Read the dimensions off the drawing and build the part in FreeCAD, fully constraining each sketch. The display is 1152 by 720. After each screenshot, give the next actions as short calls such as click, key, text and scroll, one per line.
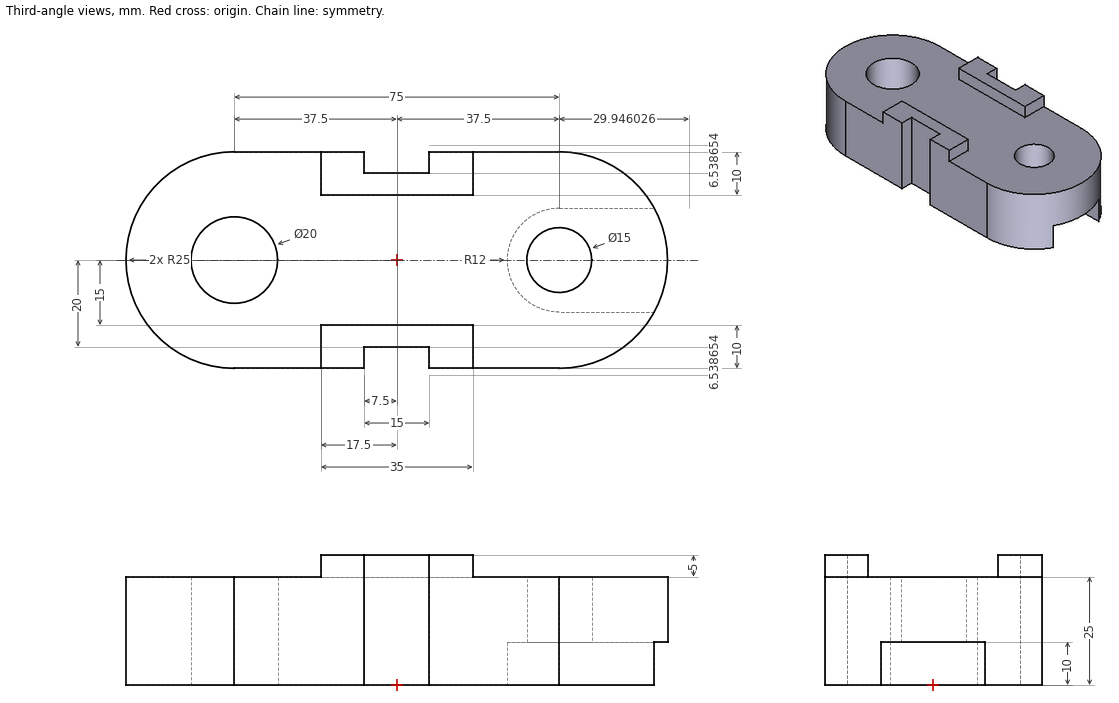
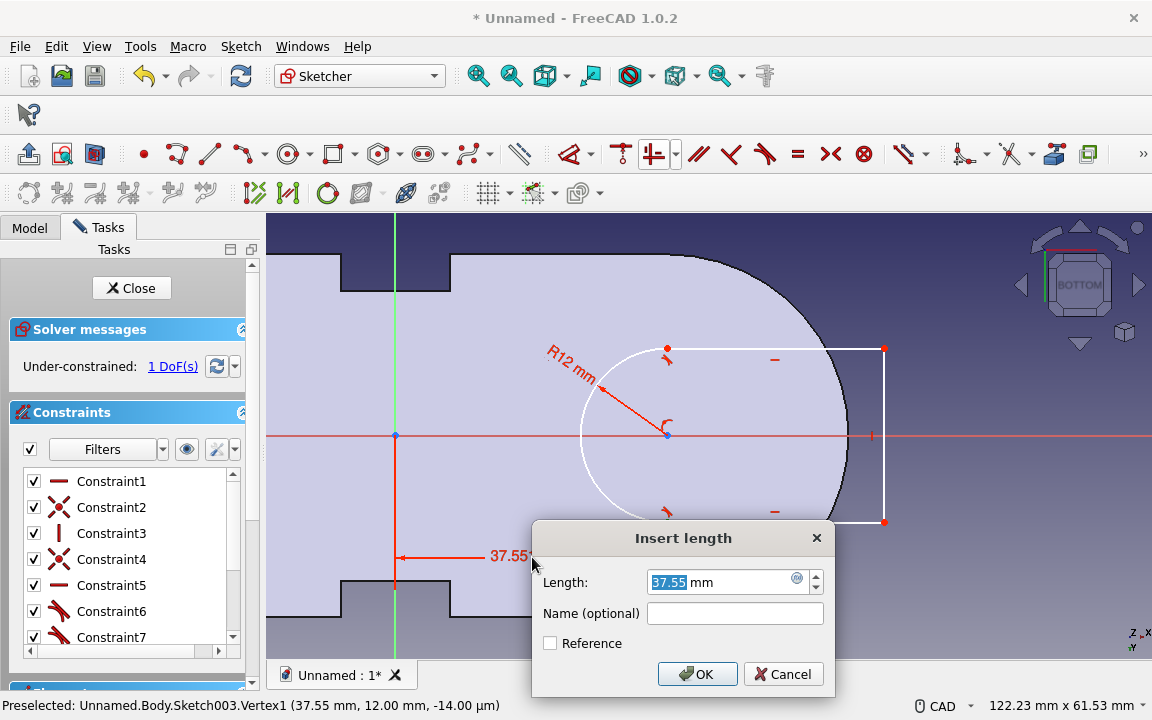
text(37.5)
key(Return)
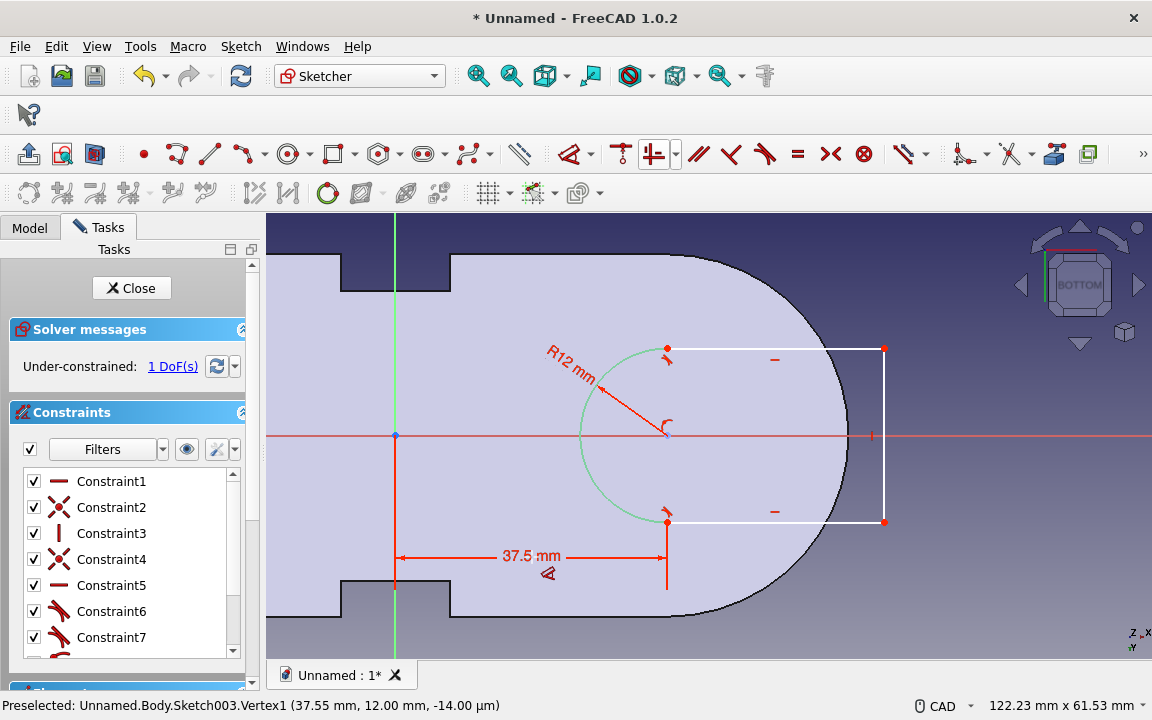
click(732, 523)
click(776, 557)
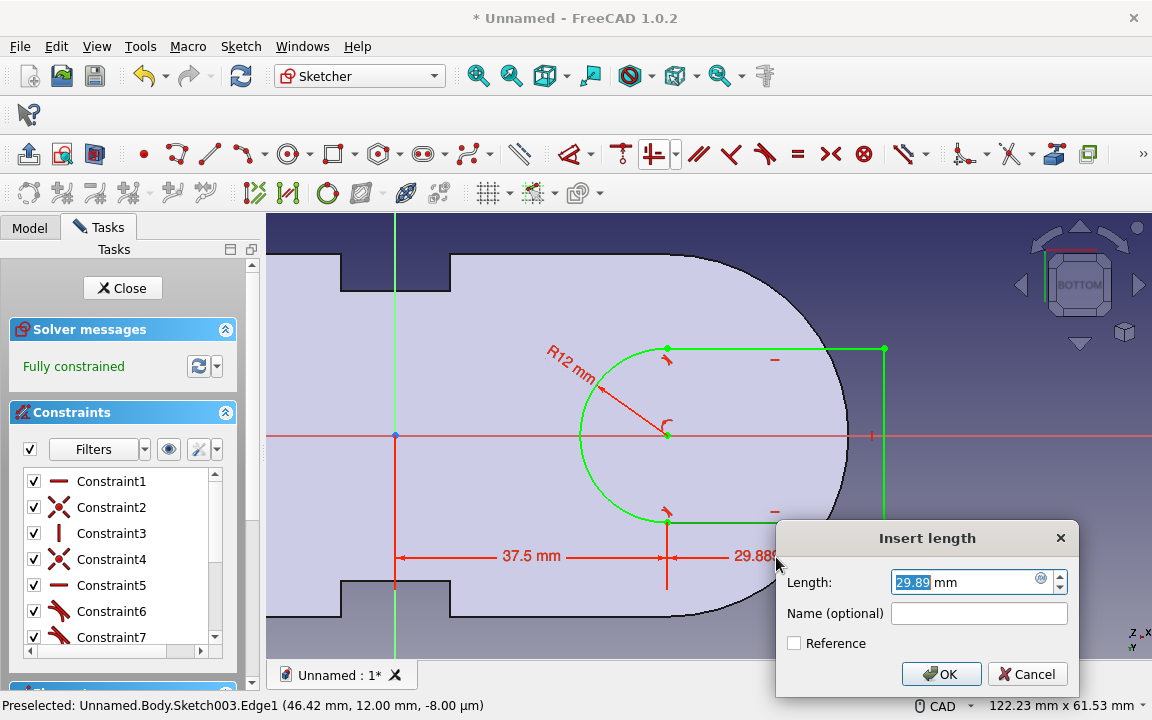
text(29.946026)
key(Return)
key(Escape)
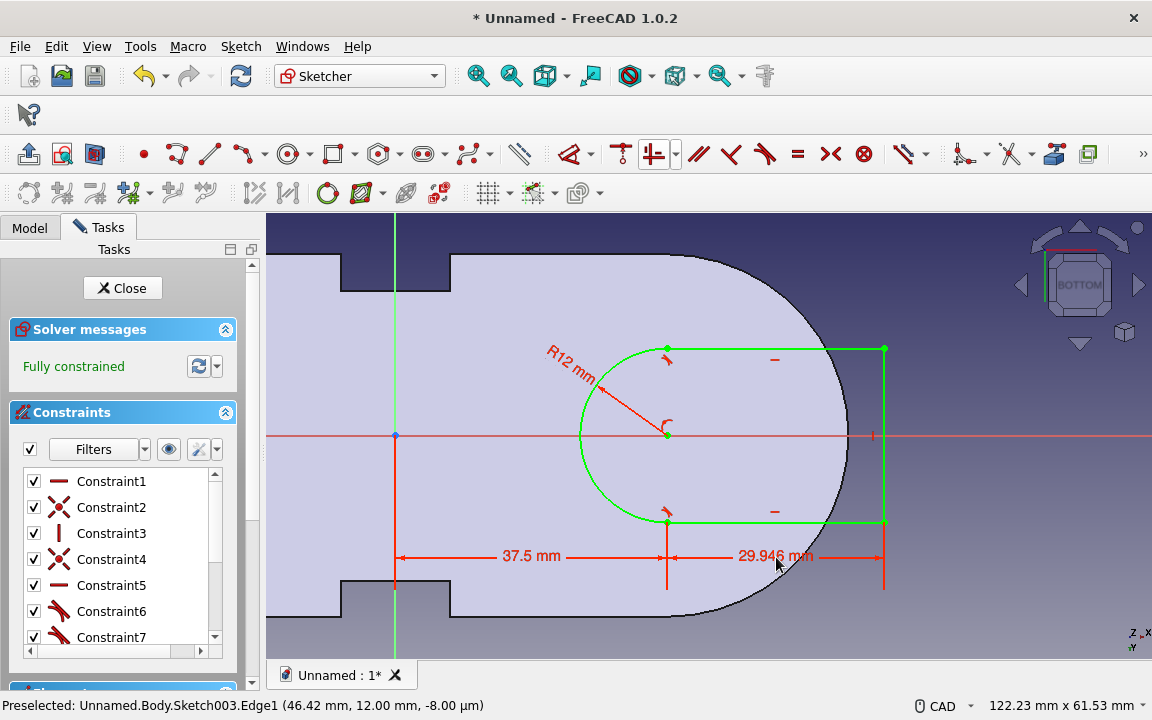
click(123, 288)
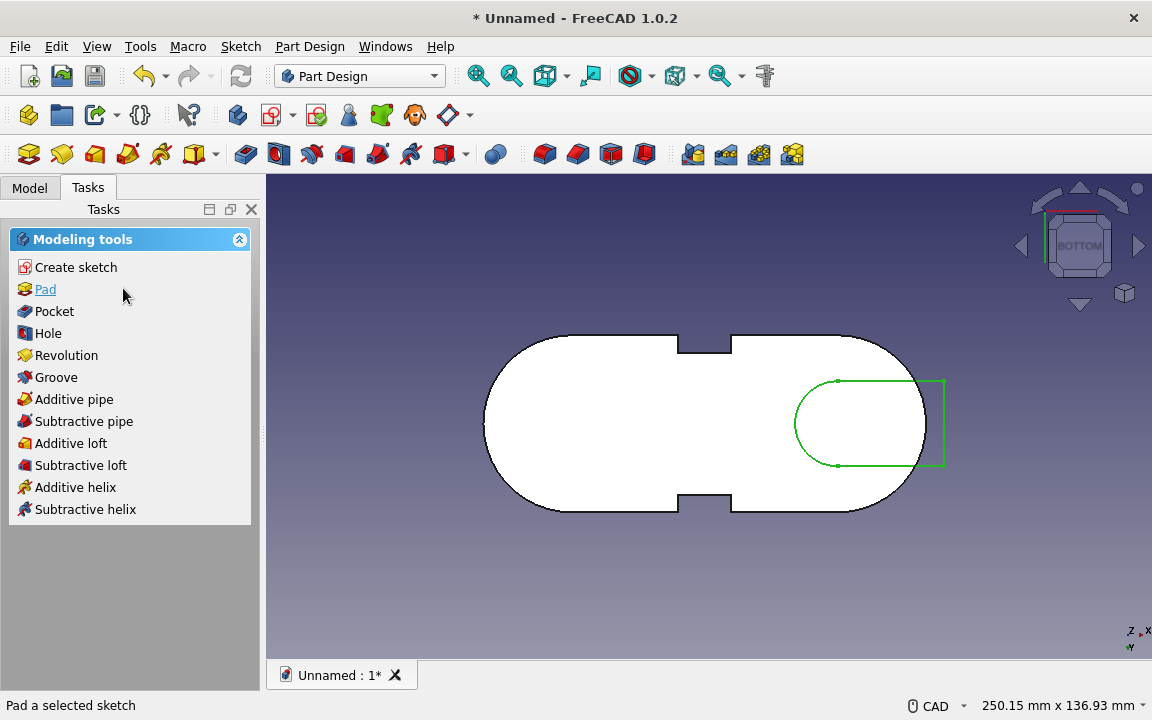
click(246, 154)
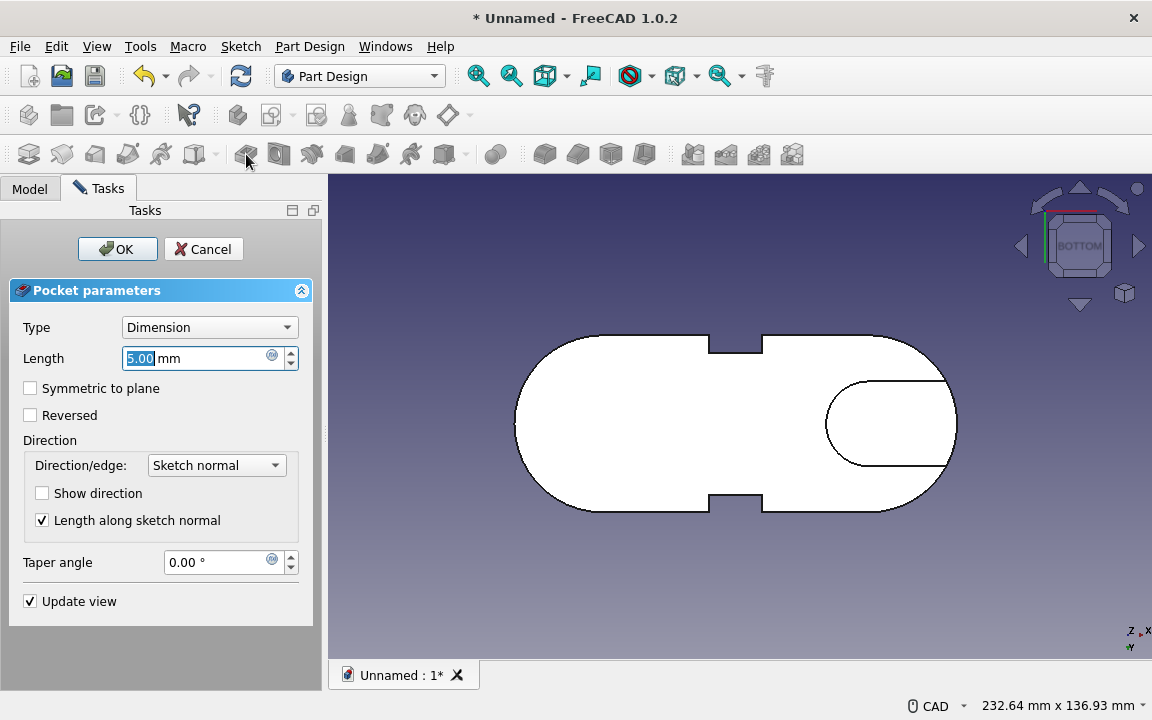
text(10)
key(Tab)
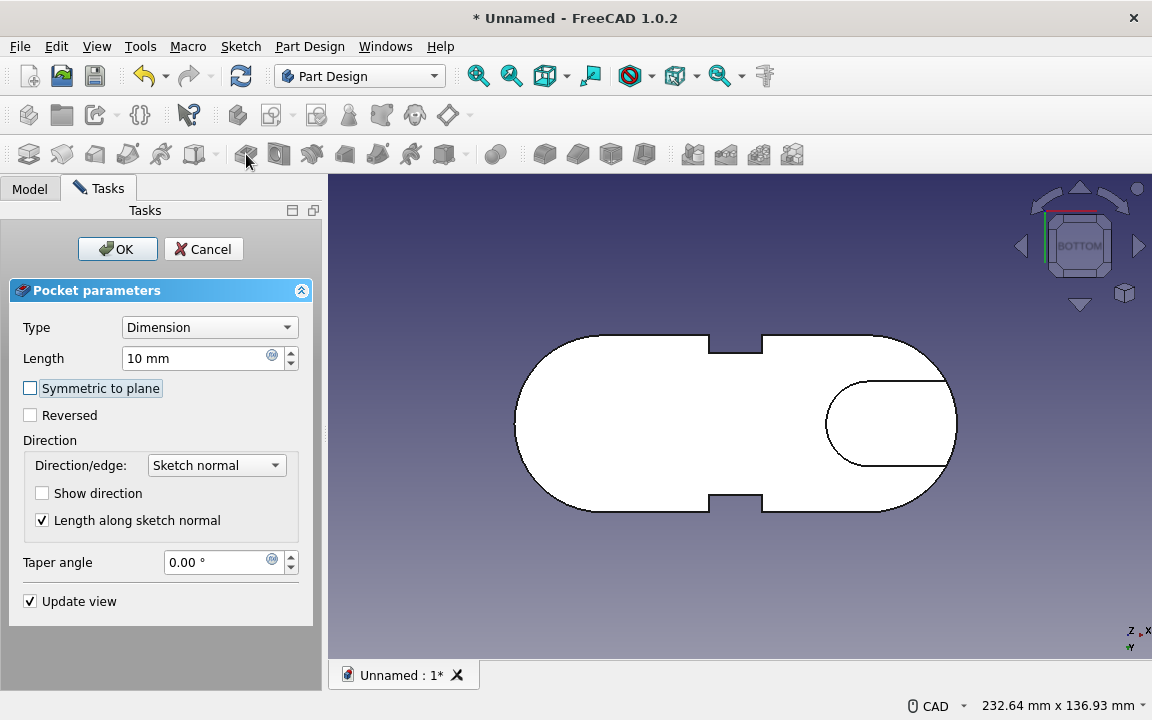
click(118, 249)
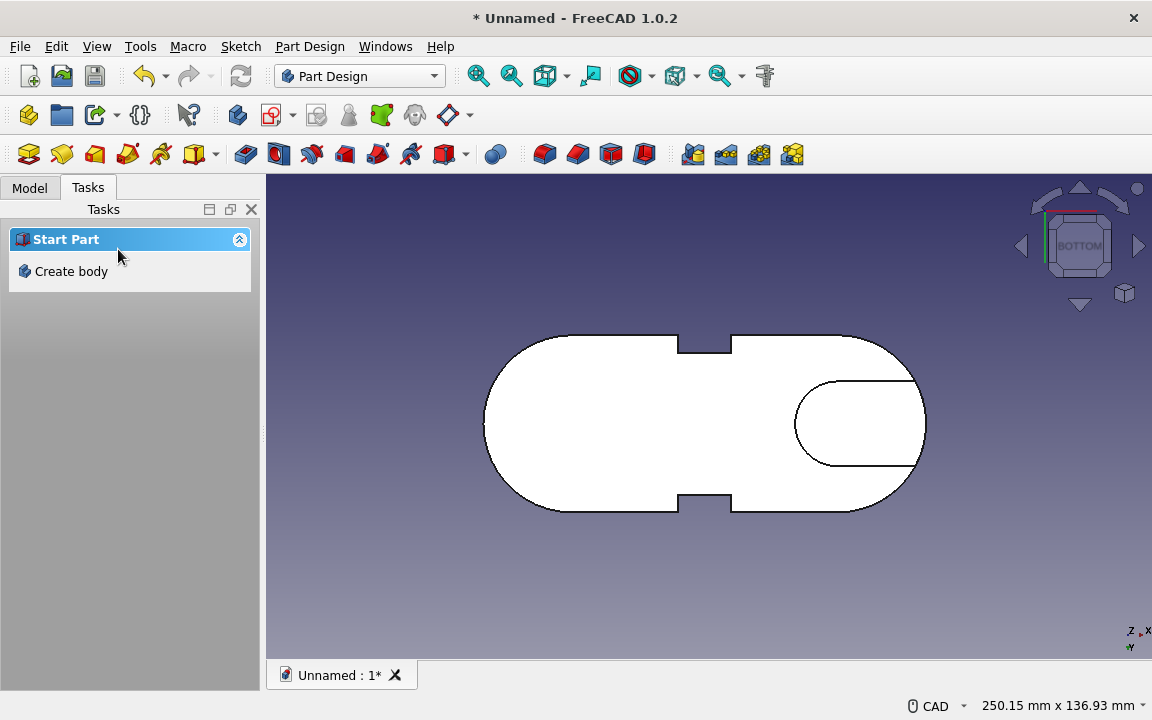
key(0)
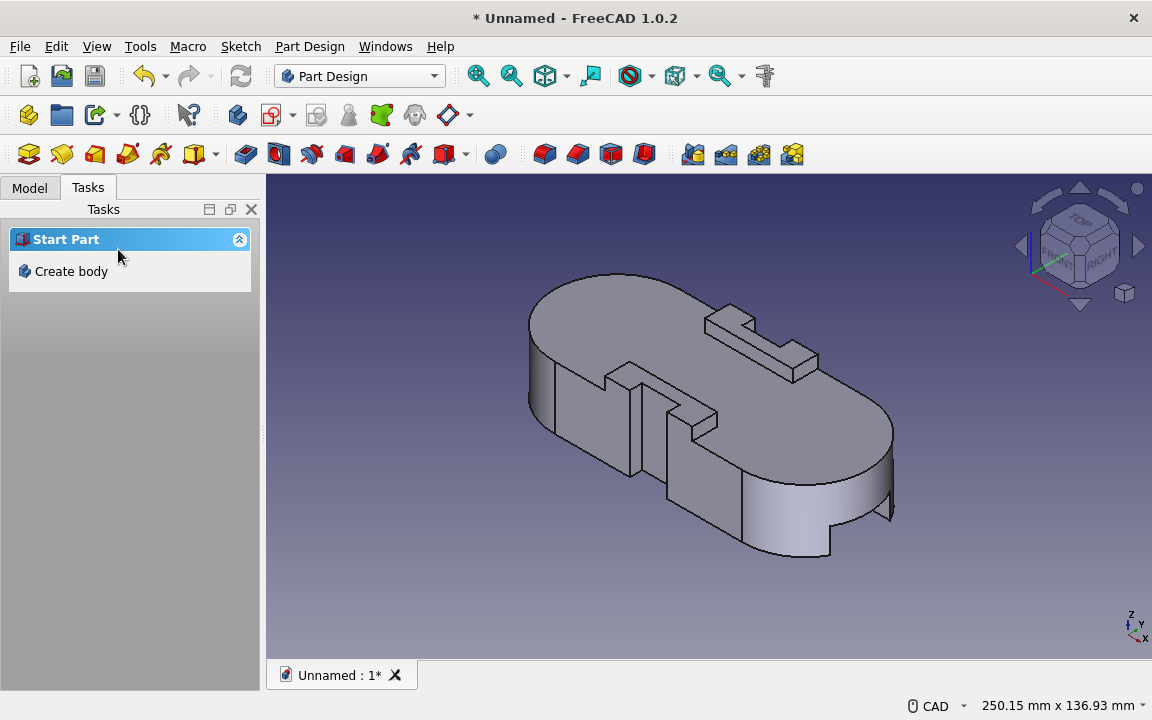
click(801, 430)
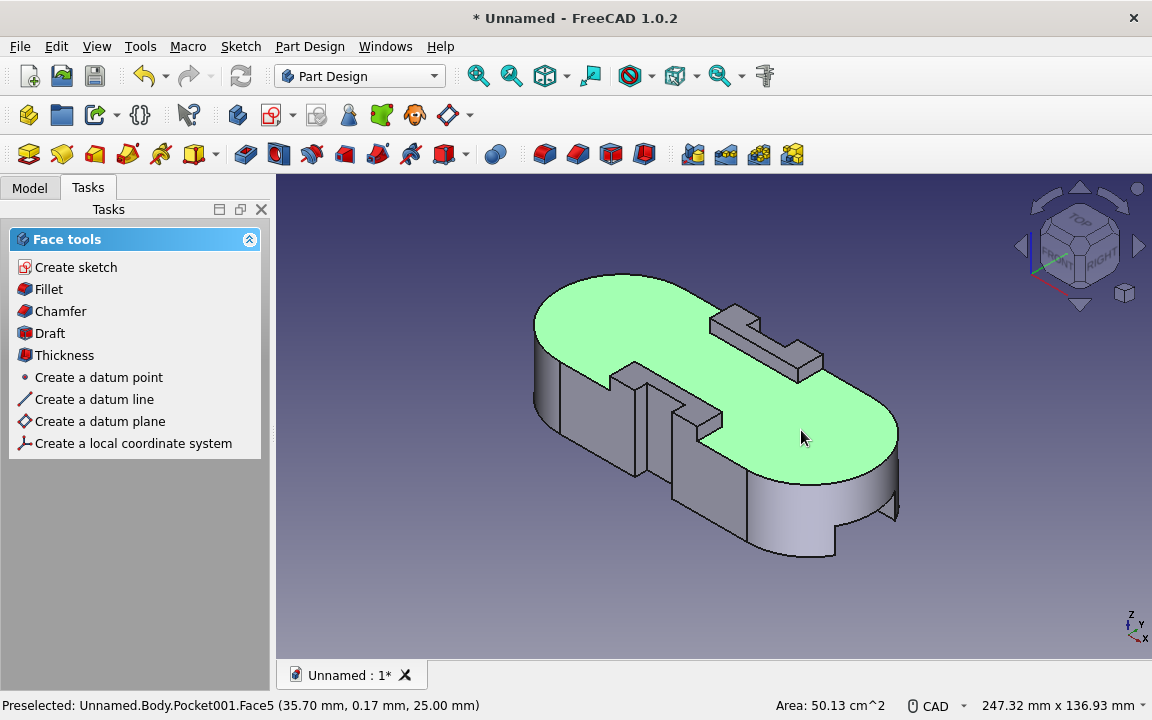
click(270, 116)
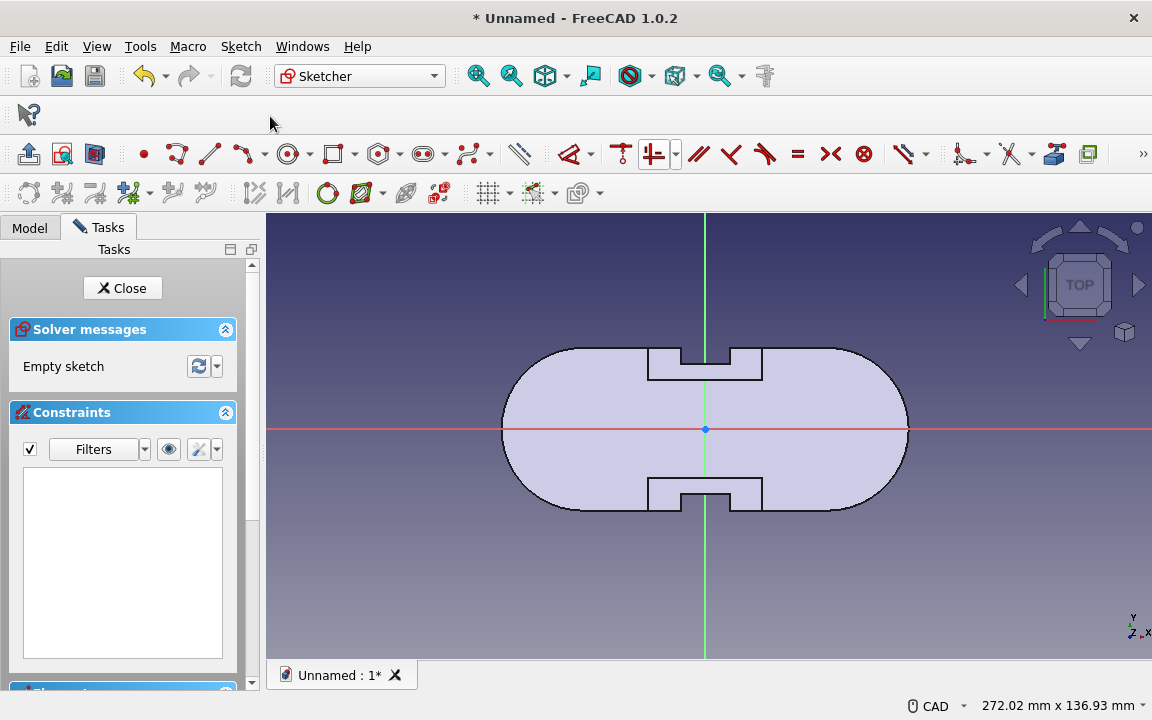
key(q)
key(s)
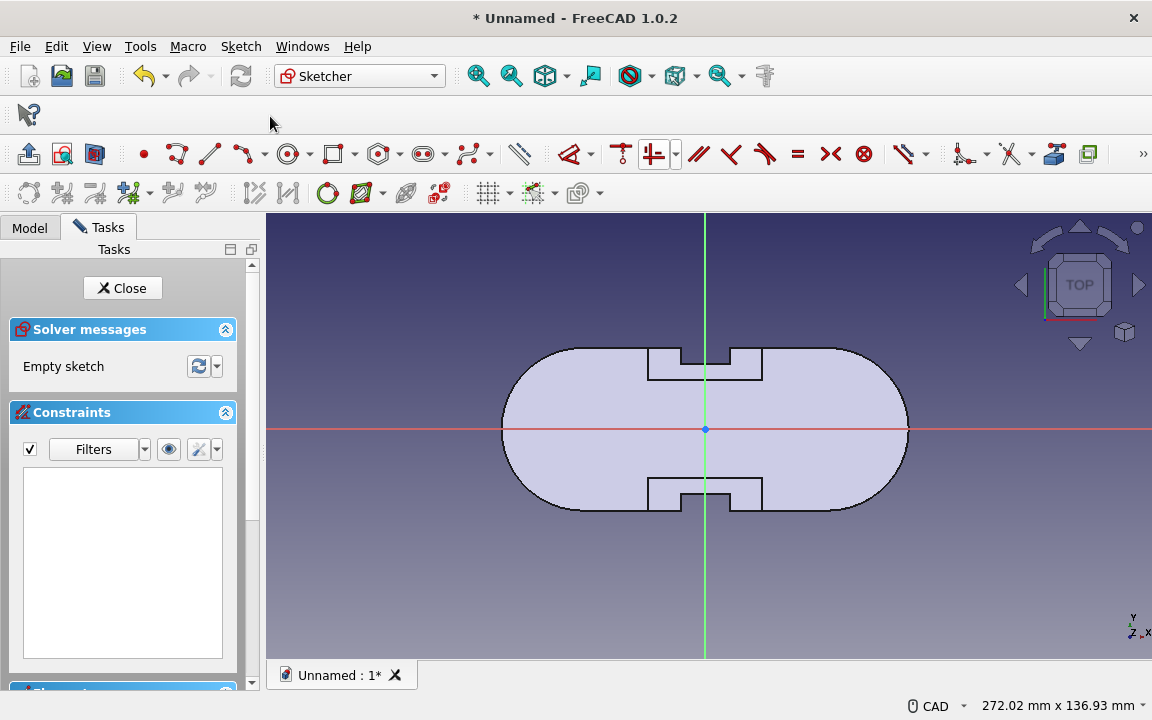
scroll(622, 426, up, 6)